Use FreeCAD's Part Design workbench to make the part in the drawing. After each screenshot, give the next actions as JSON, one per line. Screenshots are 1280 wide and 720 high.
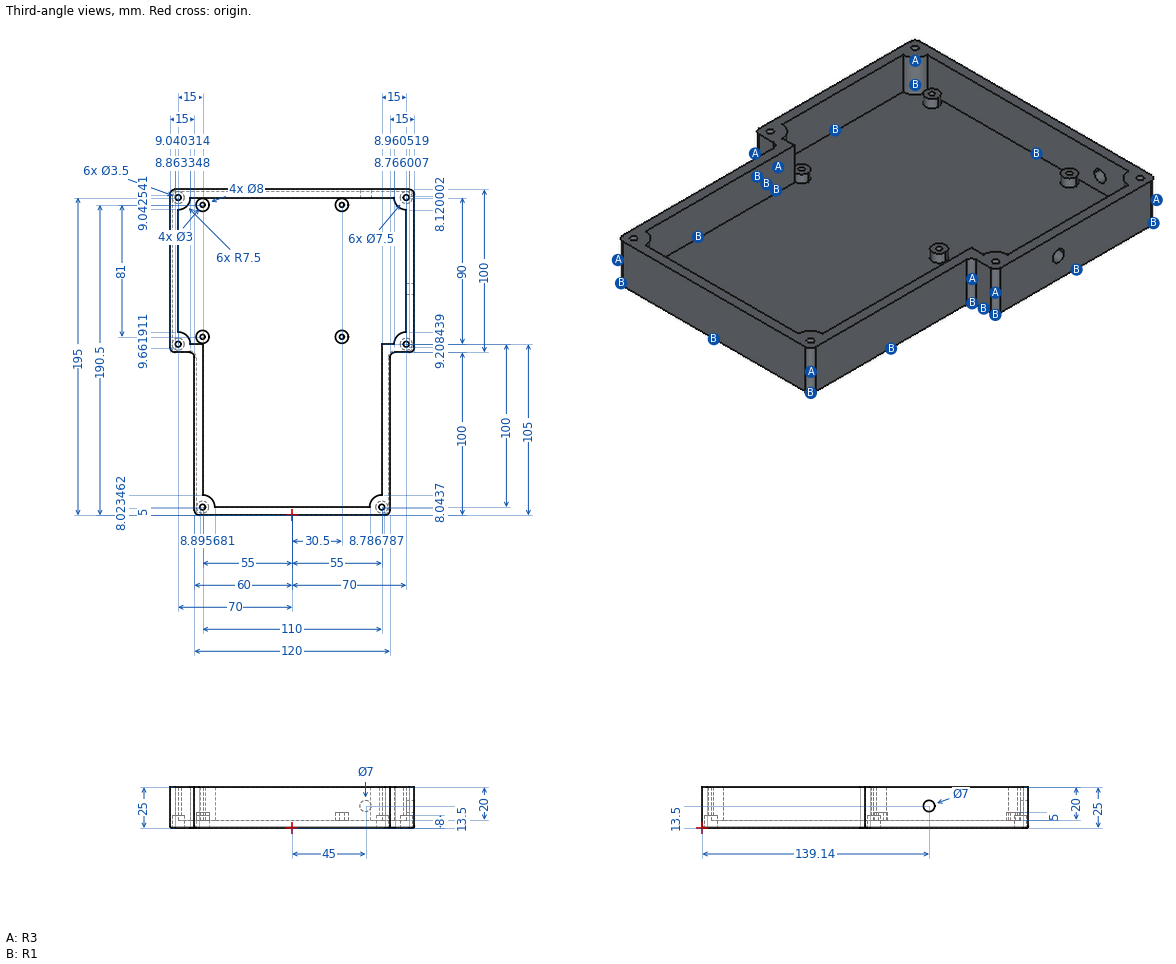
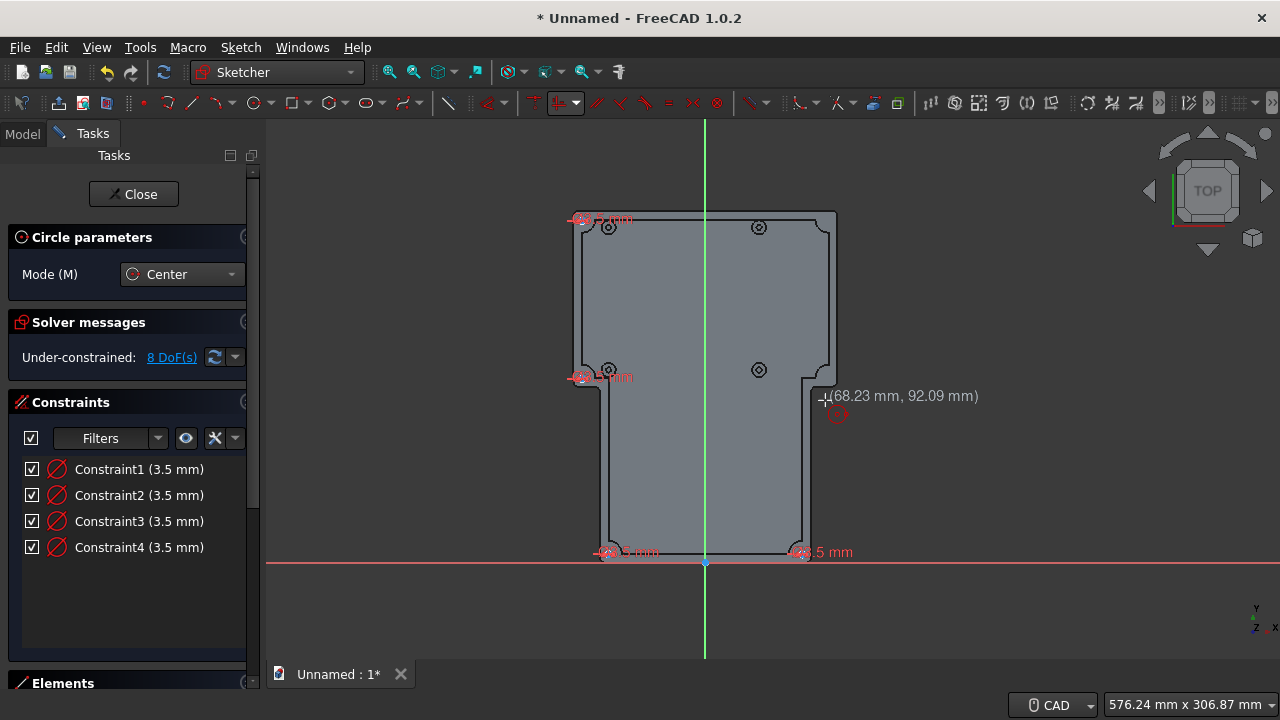
{"action": "left_click", "coordinate": [829, 378]}
{"action": "mouse_move", "coordinate": [831, 376]}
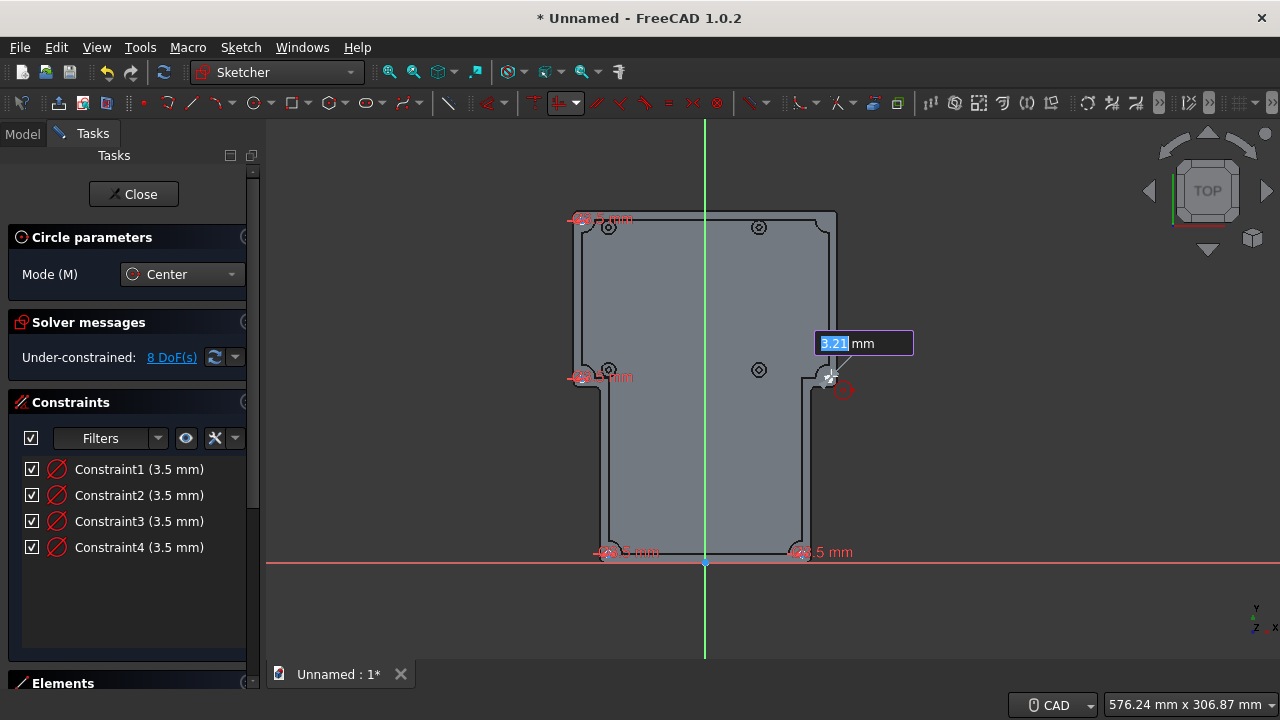
{"action": "type", "text": "3.5"}
{"action": "key", "text": "Return"}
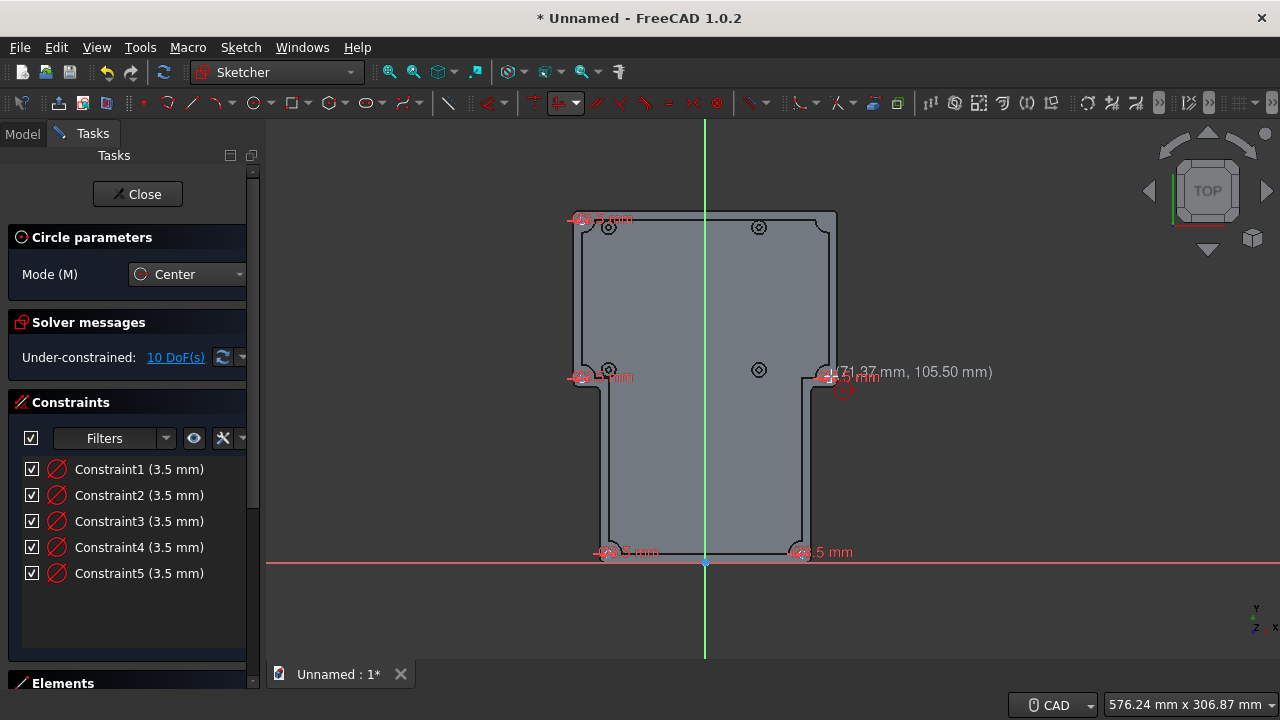
{"action": "scroll", "coordinate": [829, 220], "scroll_direction": "up", "scroll_amount": 10}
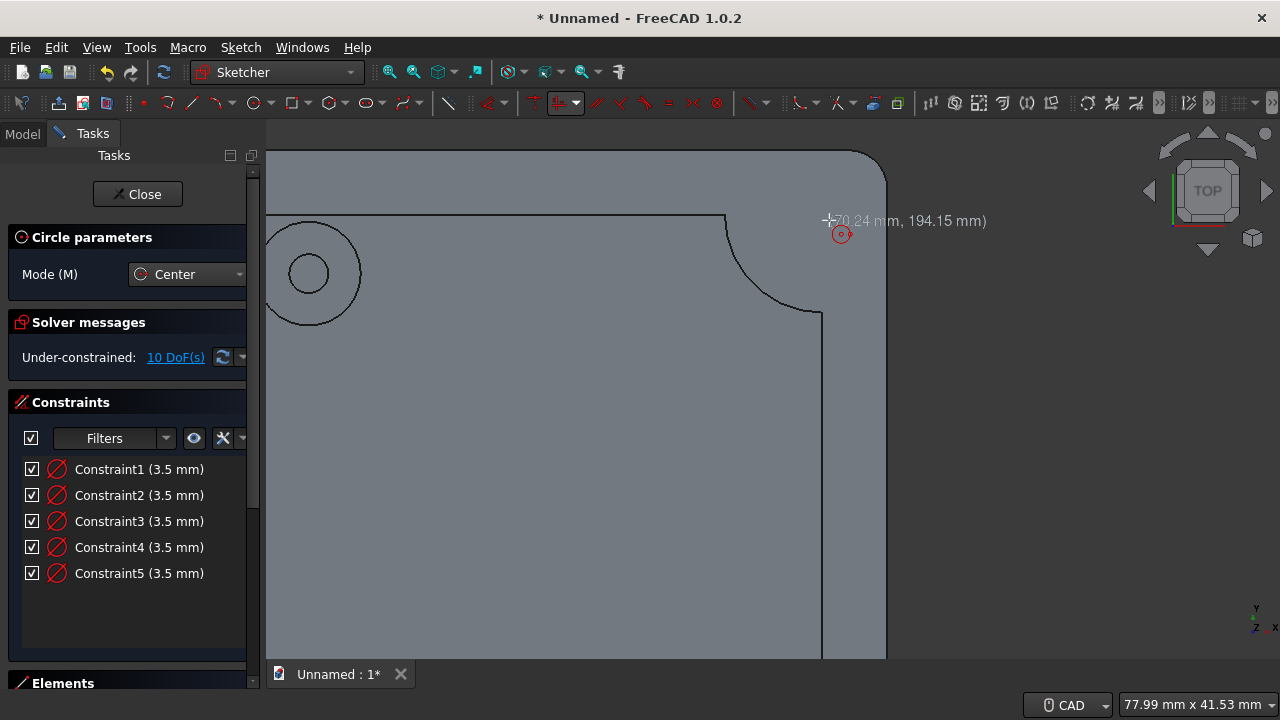
{"action": "scroll", "coordinate": [829, 220], "scroll_direction": "down", "scroll_amount": 10}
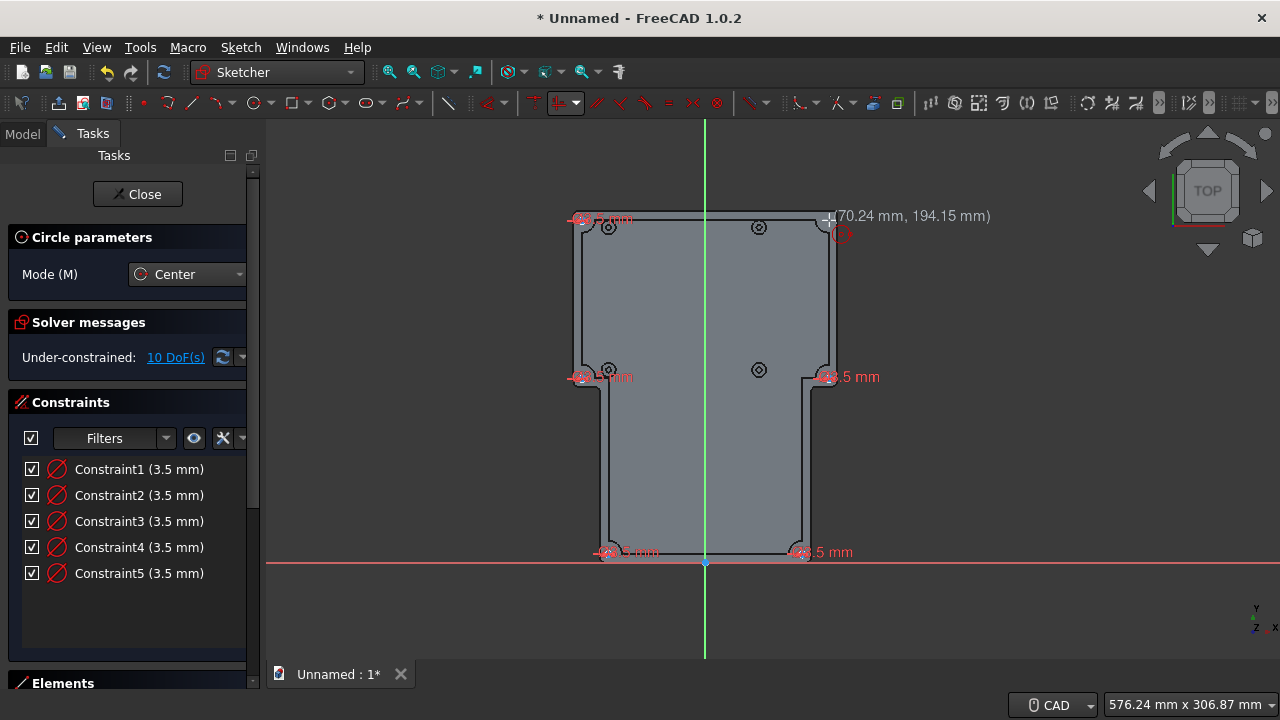
{"action": "left_click", "coordinate": [829, 220]}
{"action": "mouse_move", "coordinate": [831, 217]}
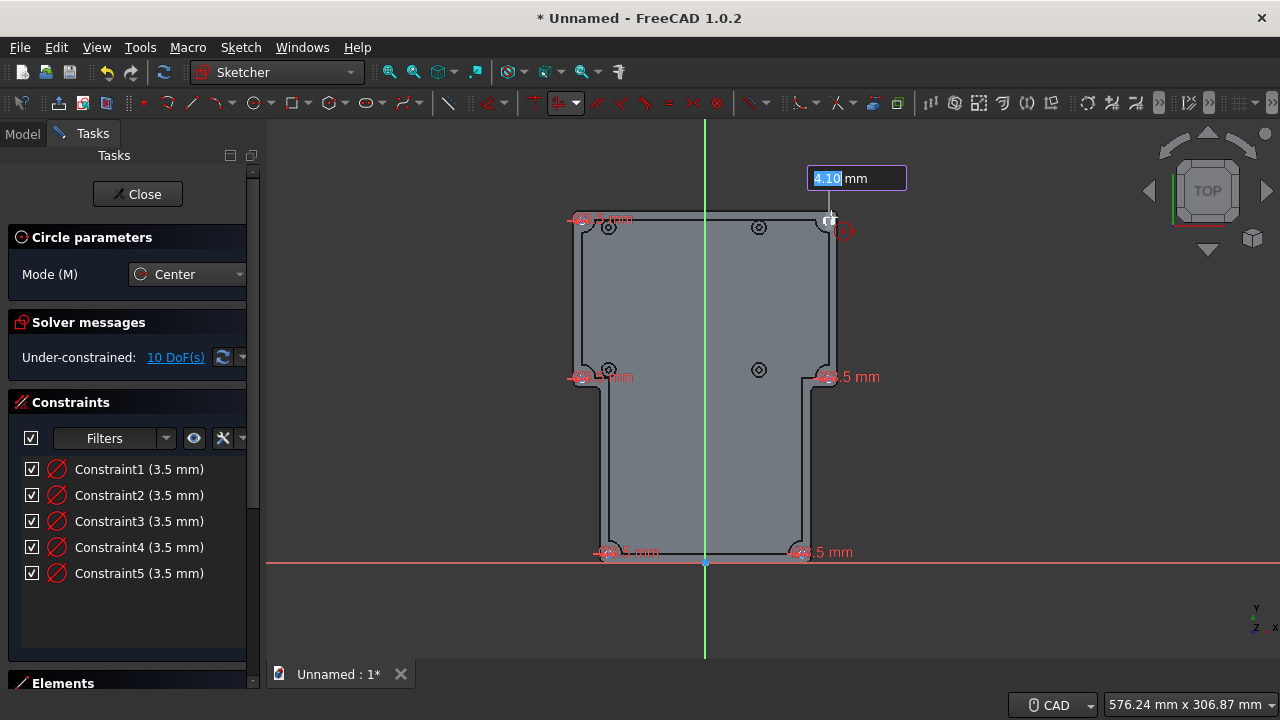
{"action": "type", "text": "3.5"}
{"action": "key", "text": "Return"}
{"action": "key", "text": "Escape"}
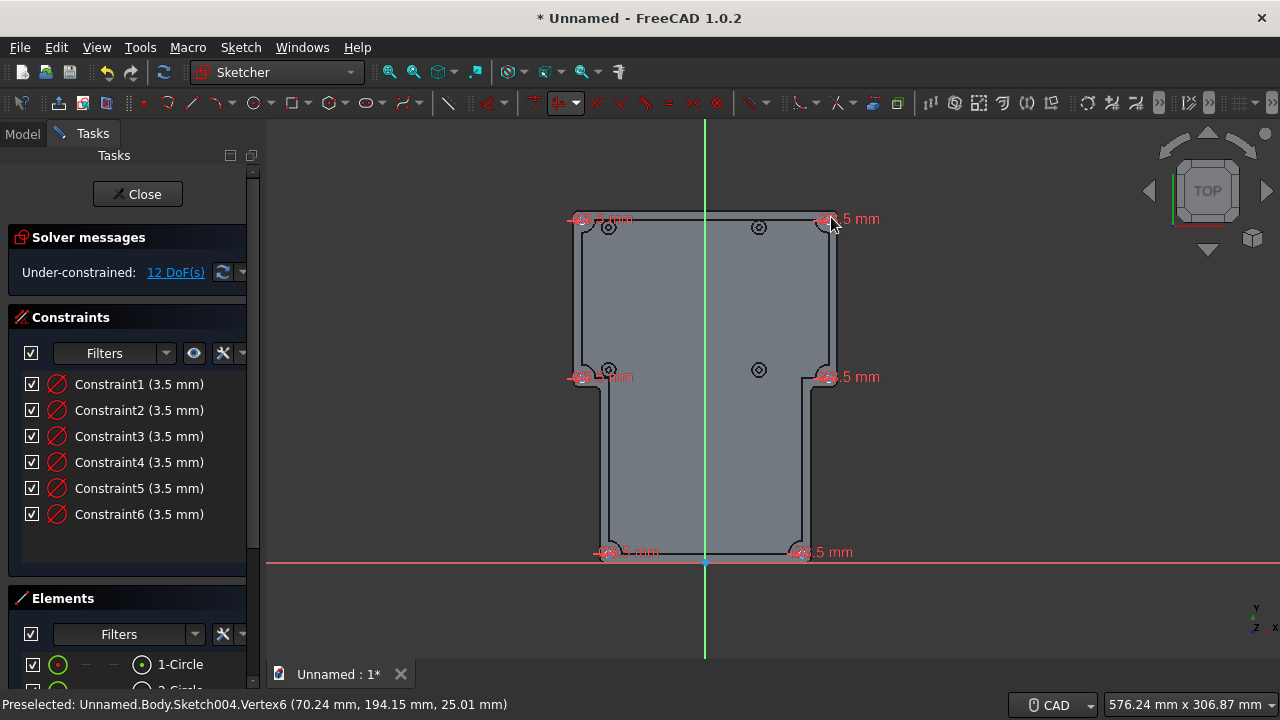
{"action": "left_click", "coordinate": [582, 221]}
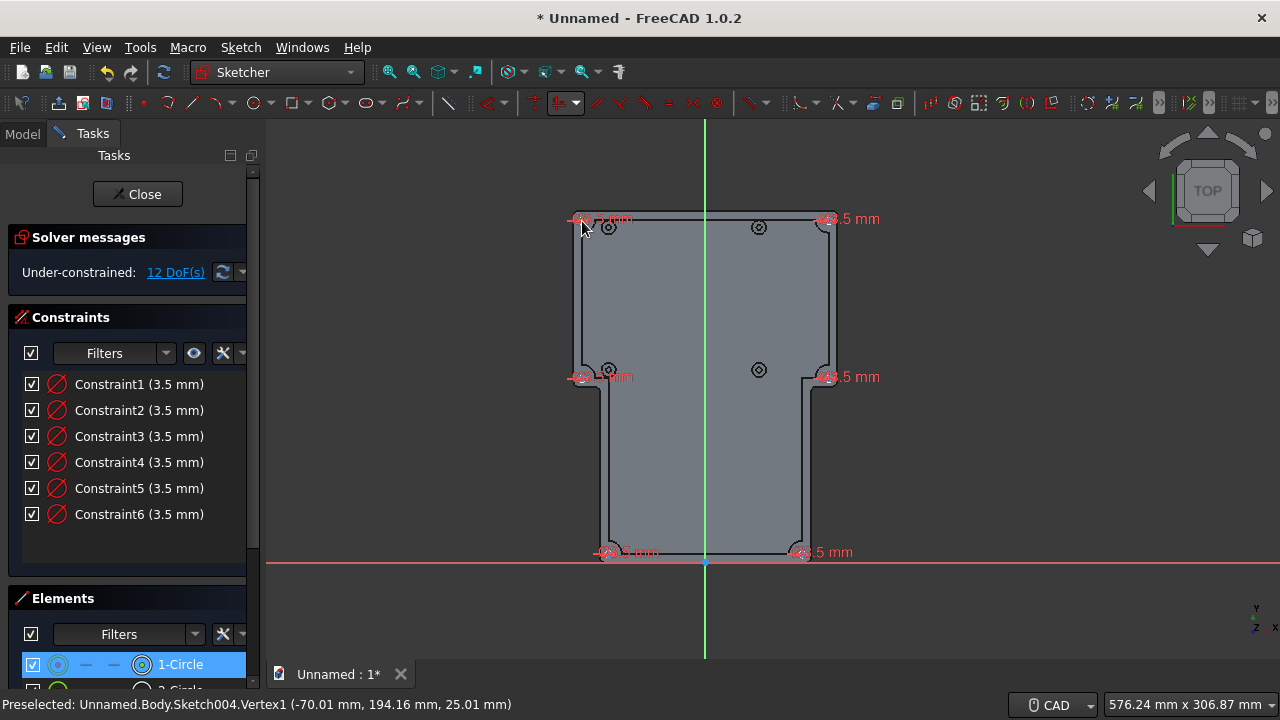
{"action": "left_click", "coordinate": [582, 379]}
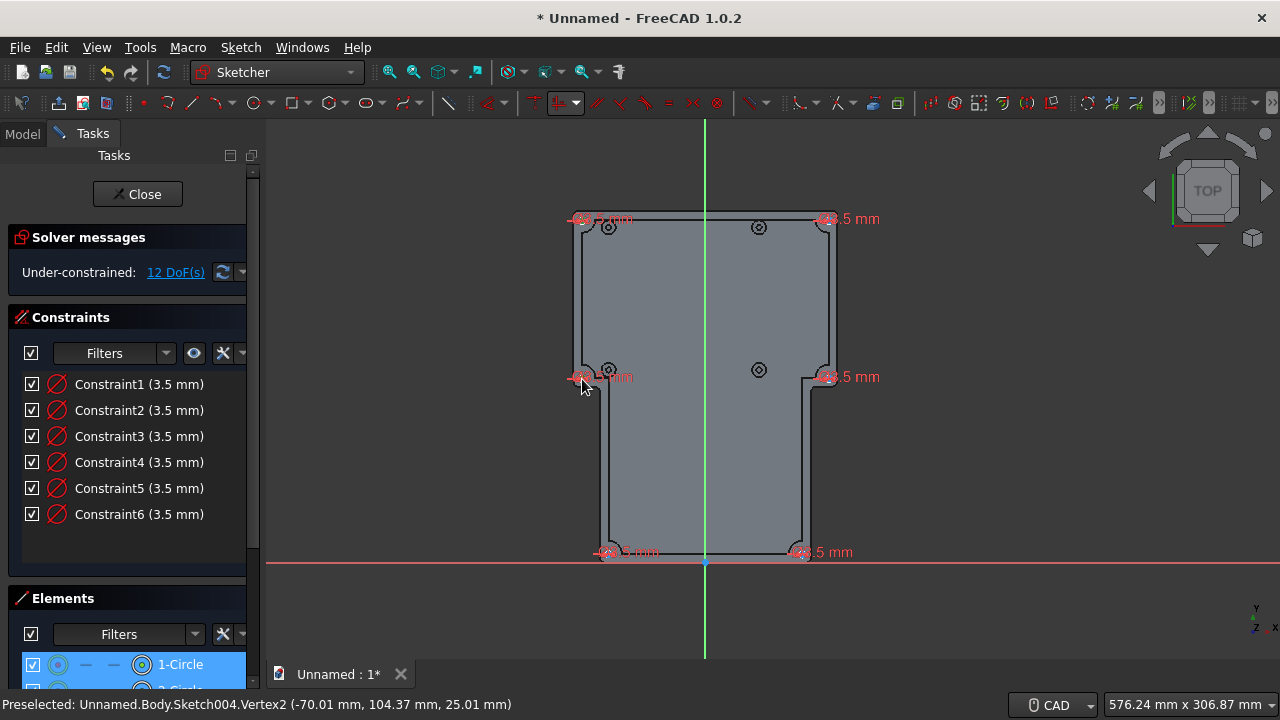
{"action": "key", "text": "v"}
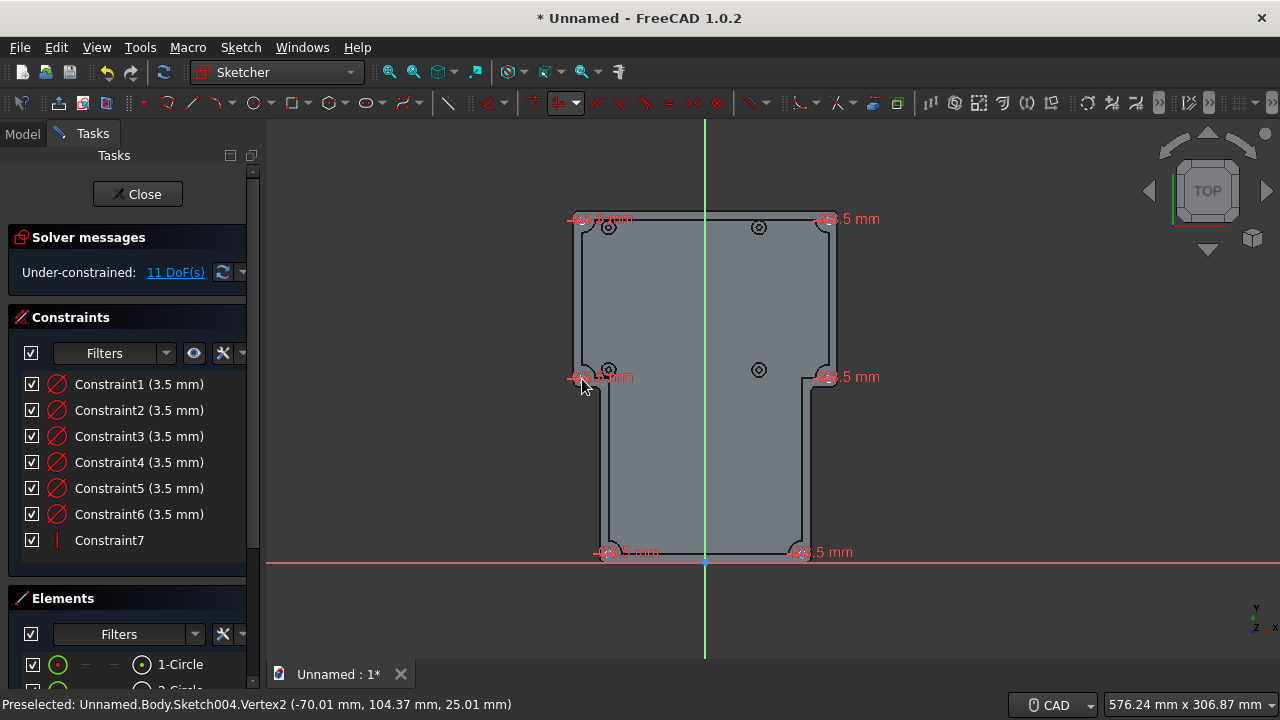
{"action": "left_click", "coordinate": [608, 554]}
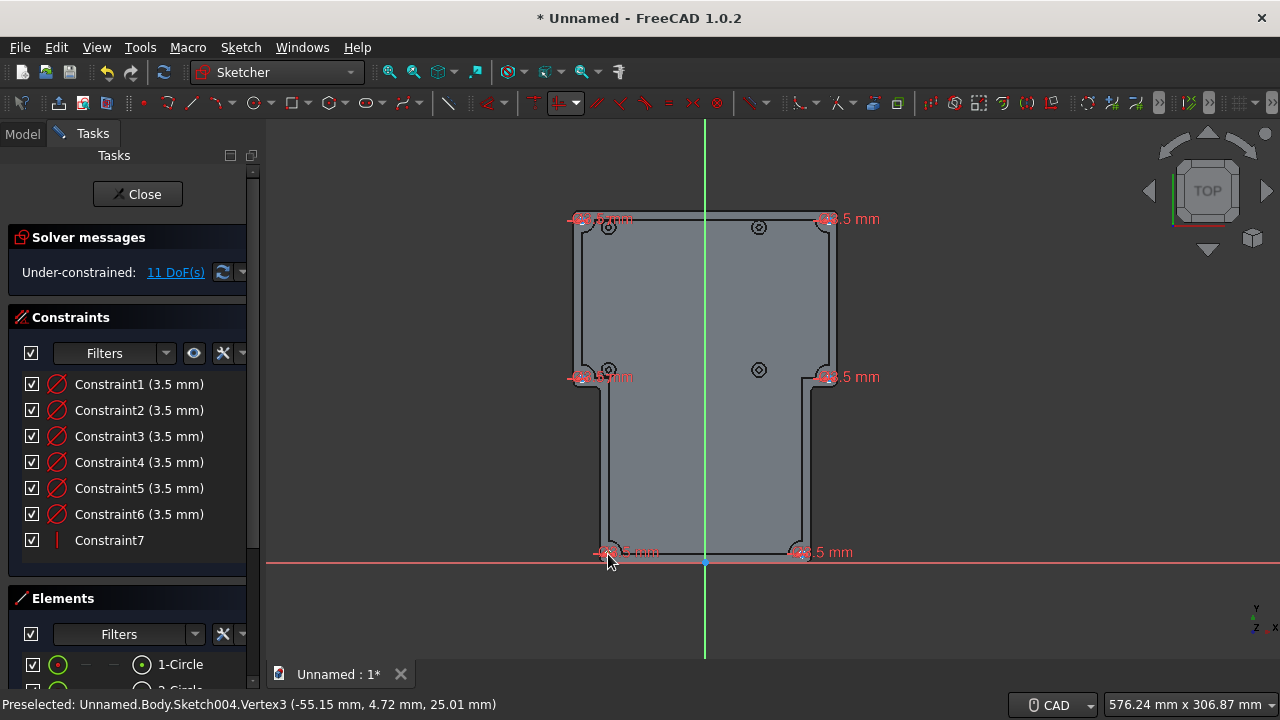
{"action": "left_click", "coordinate": [802, 554]}